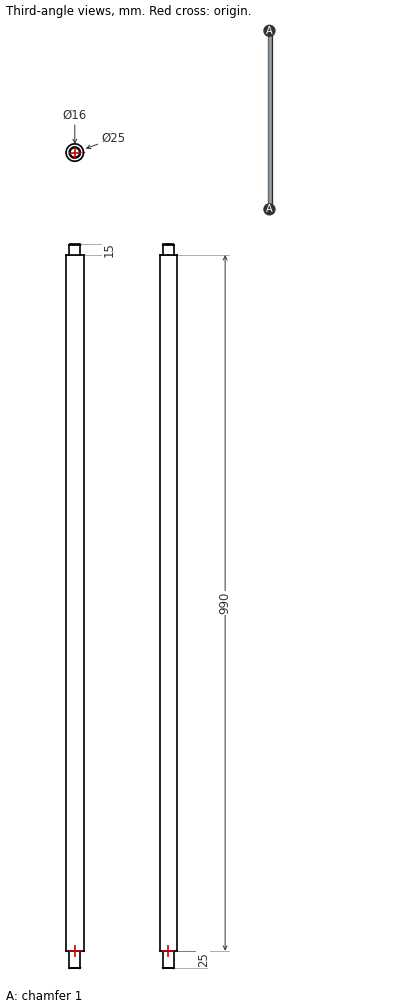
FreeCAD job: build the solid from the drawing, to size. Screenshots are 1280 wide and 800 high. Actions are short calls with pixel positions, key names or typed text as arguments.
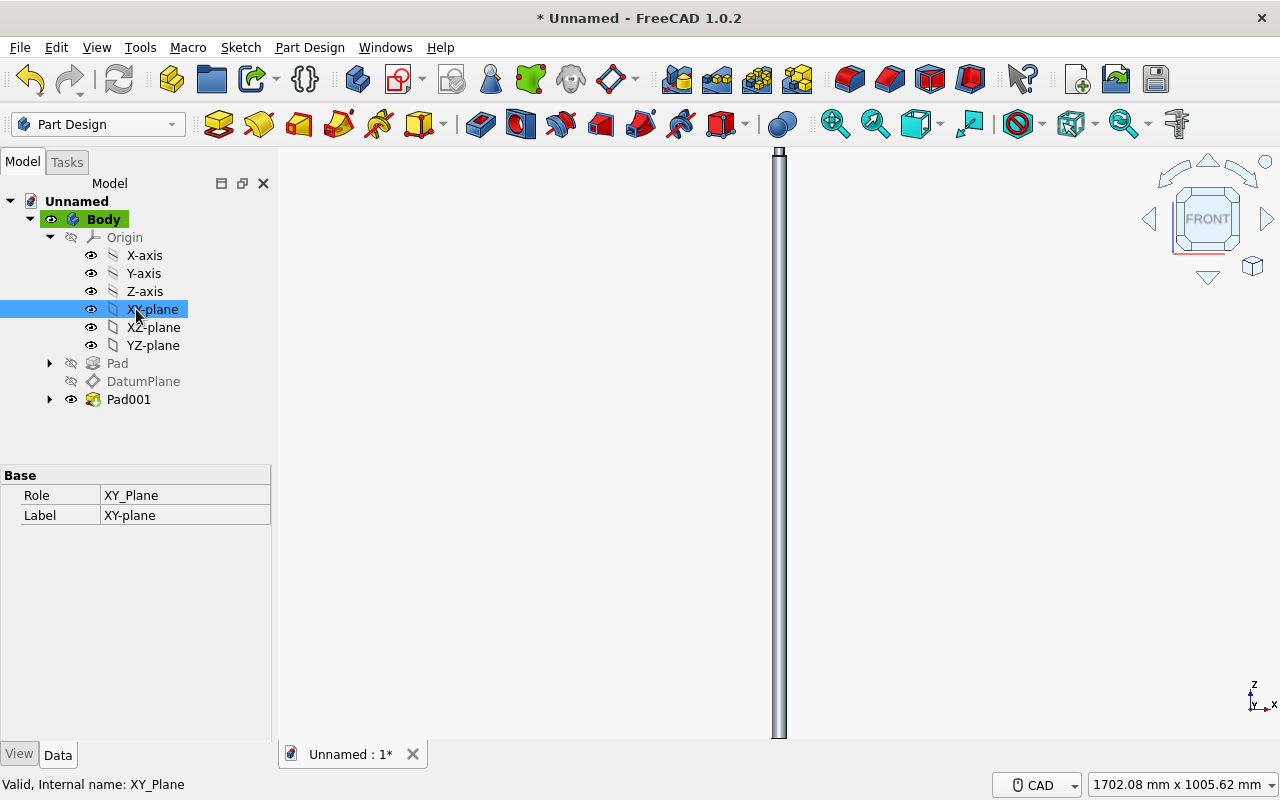
click(612, 80)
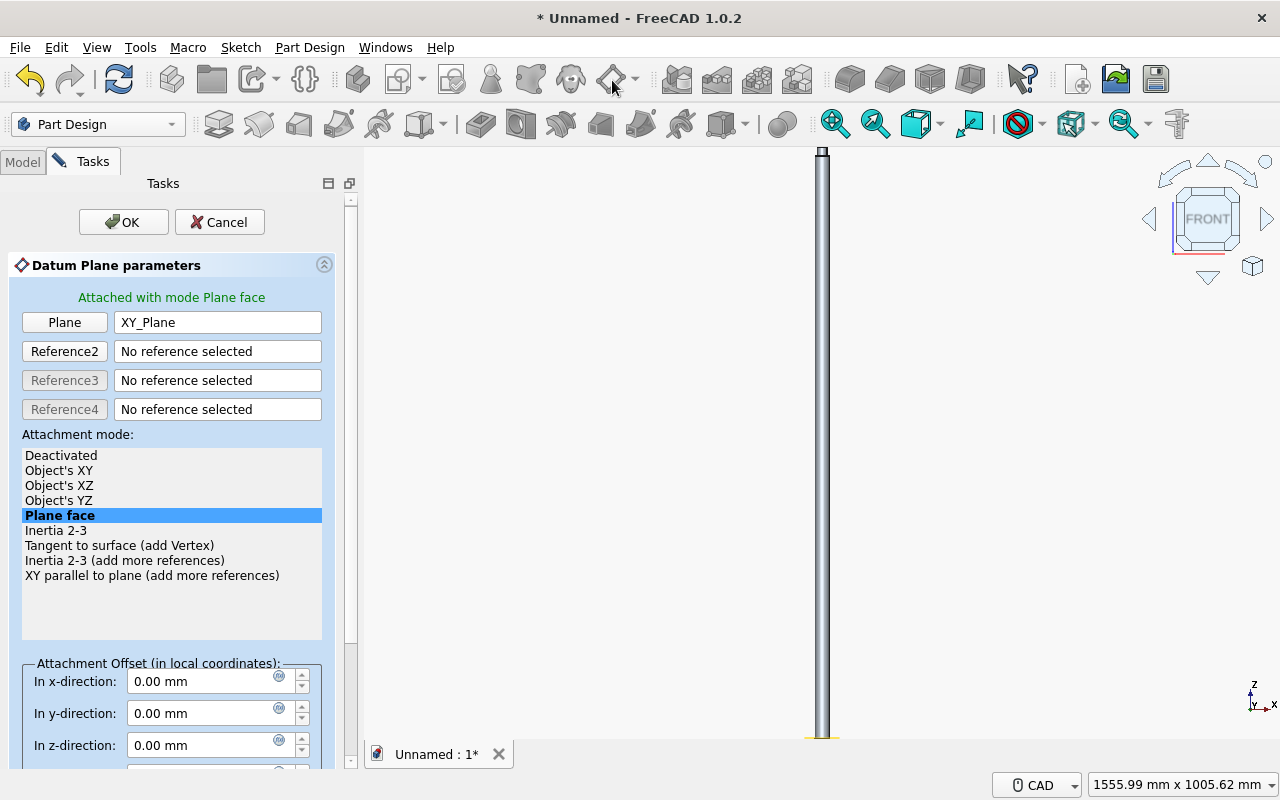
triple_click(210, 745)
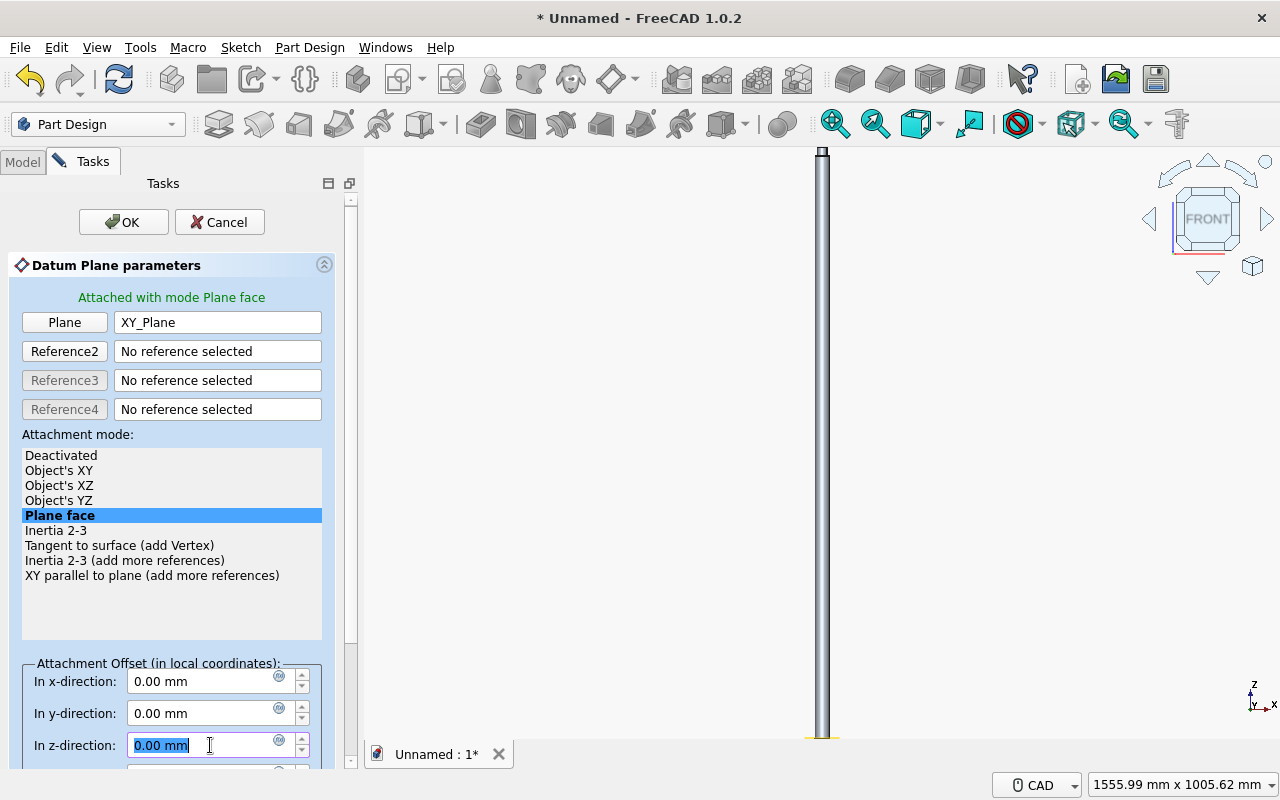
text(-25)
key(Tab)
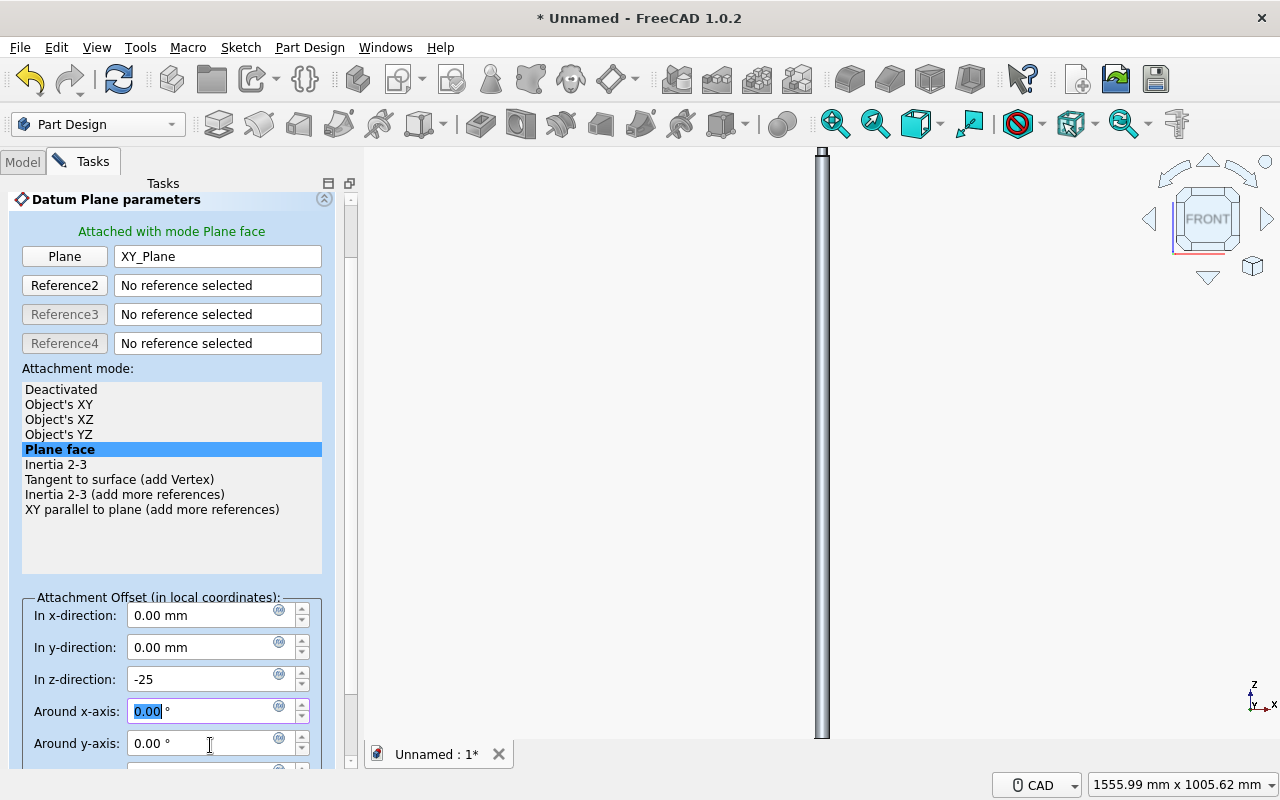
scroll(351, 480, up, 2)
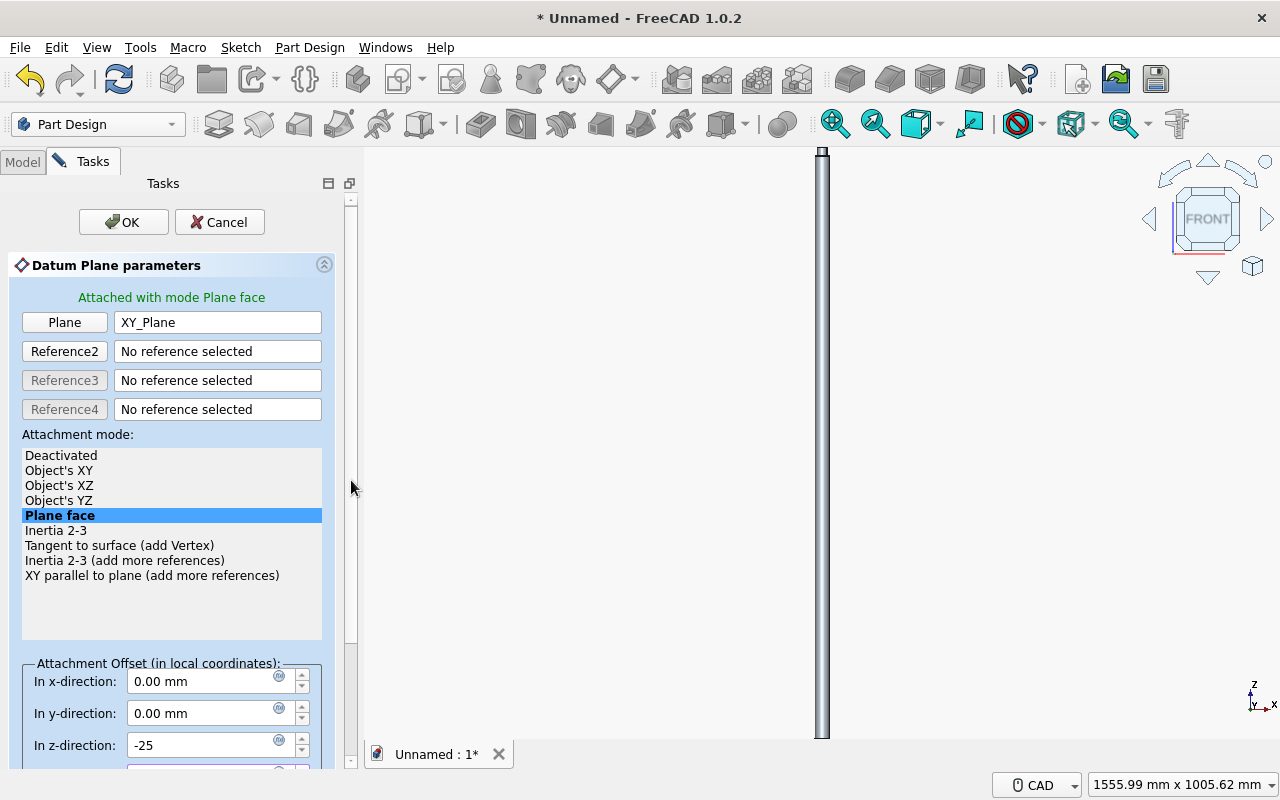
click(124, 222)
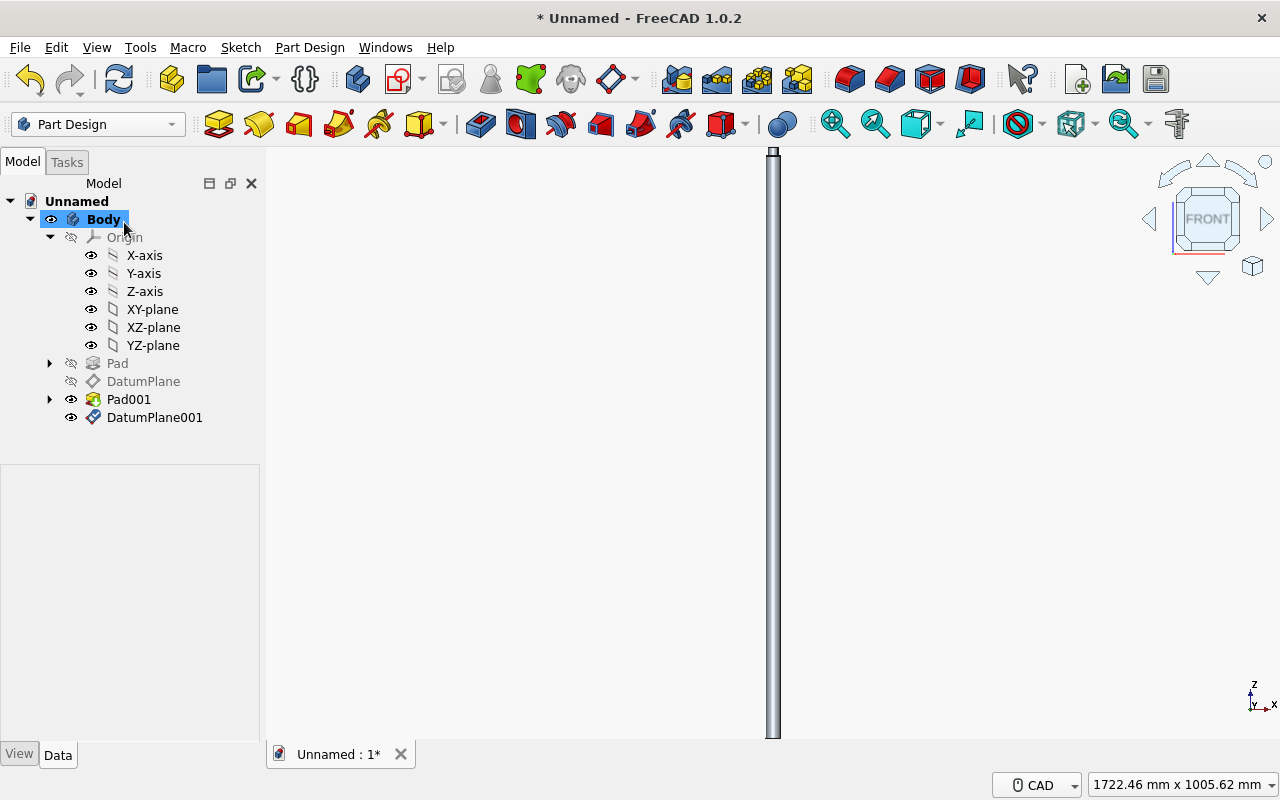
click(116, 417)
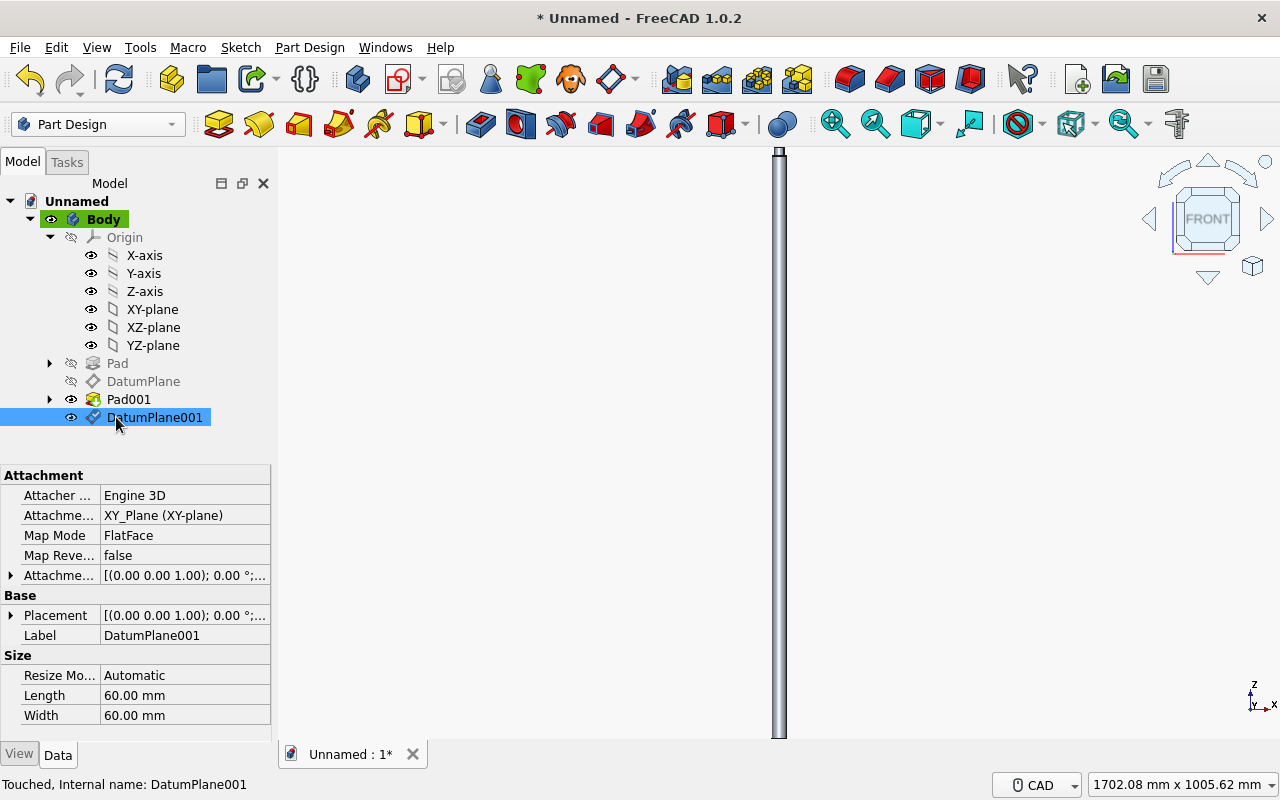
click(398, 80)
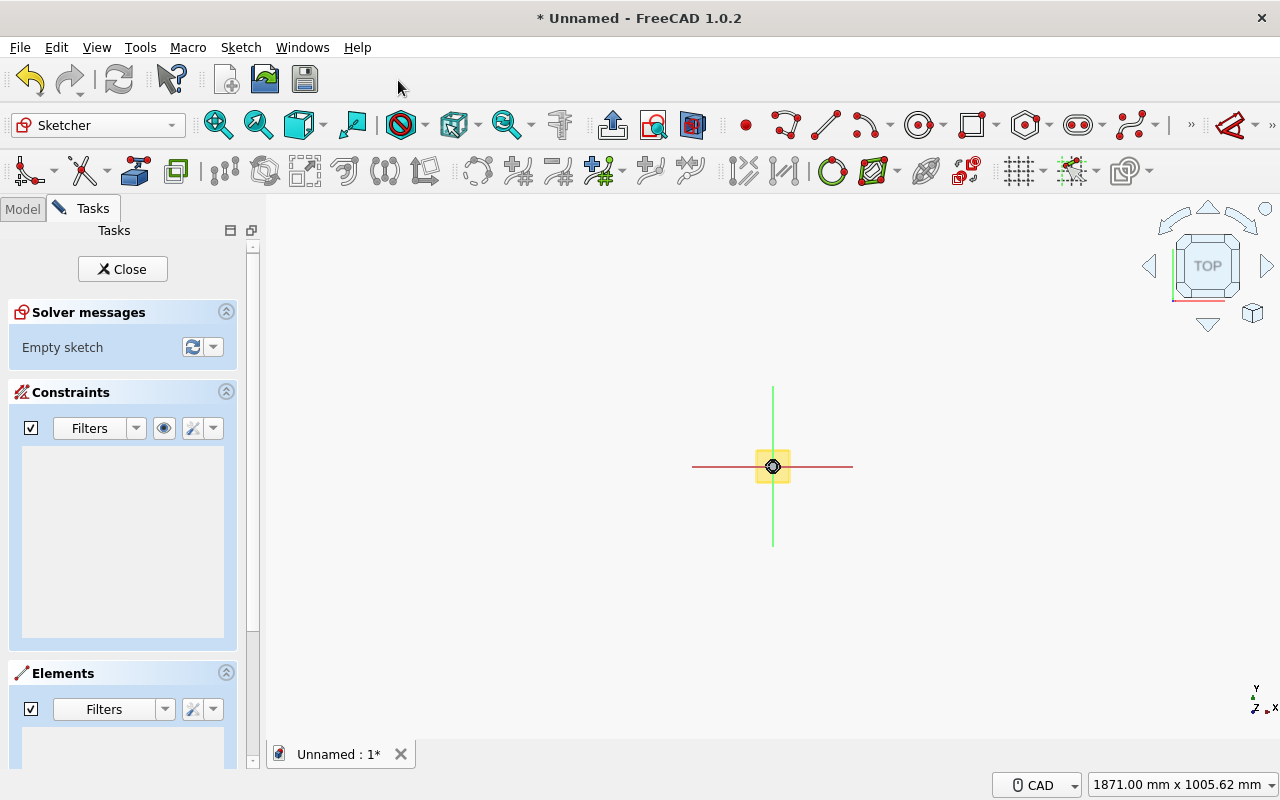
click(694, 126)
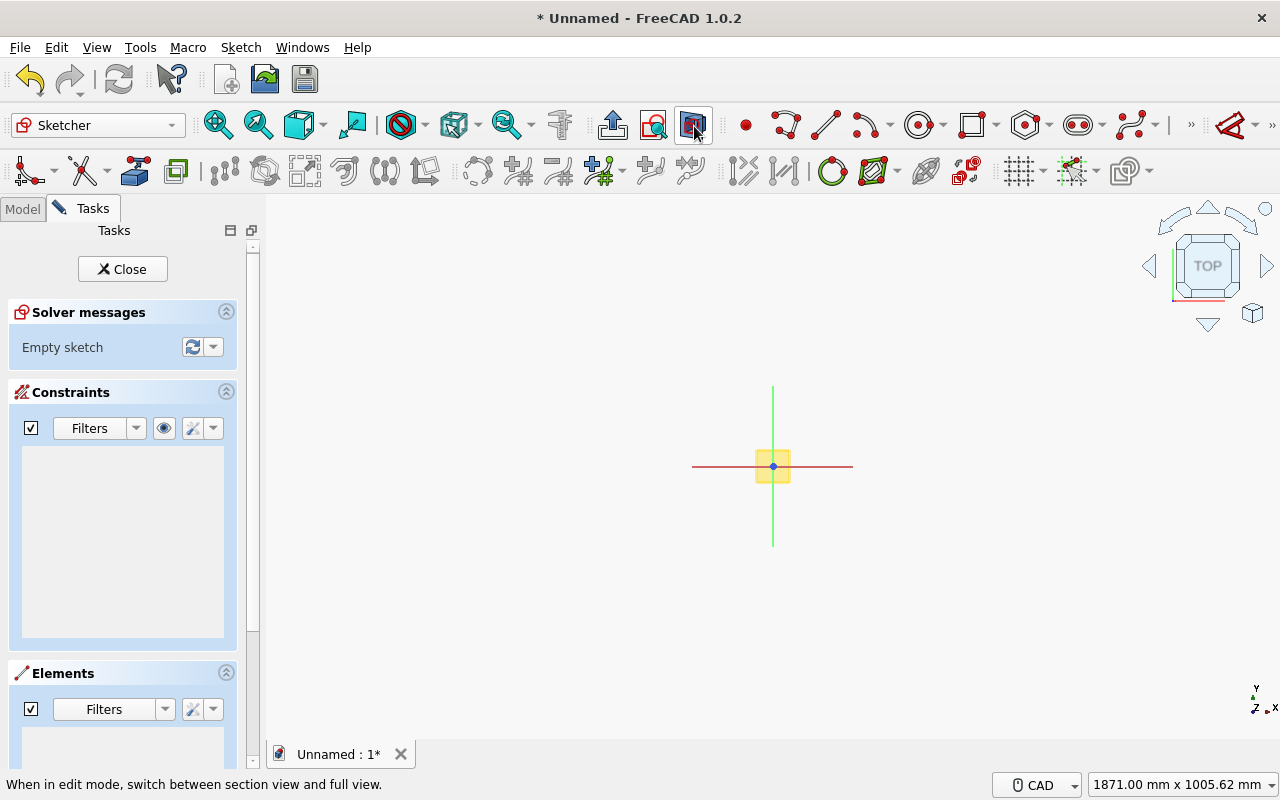
scroll(777, 466, up, 15)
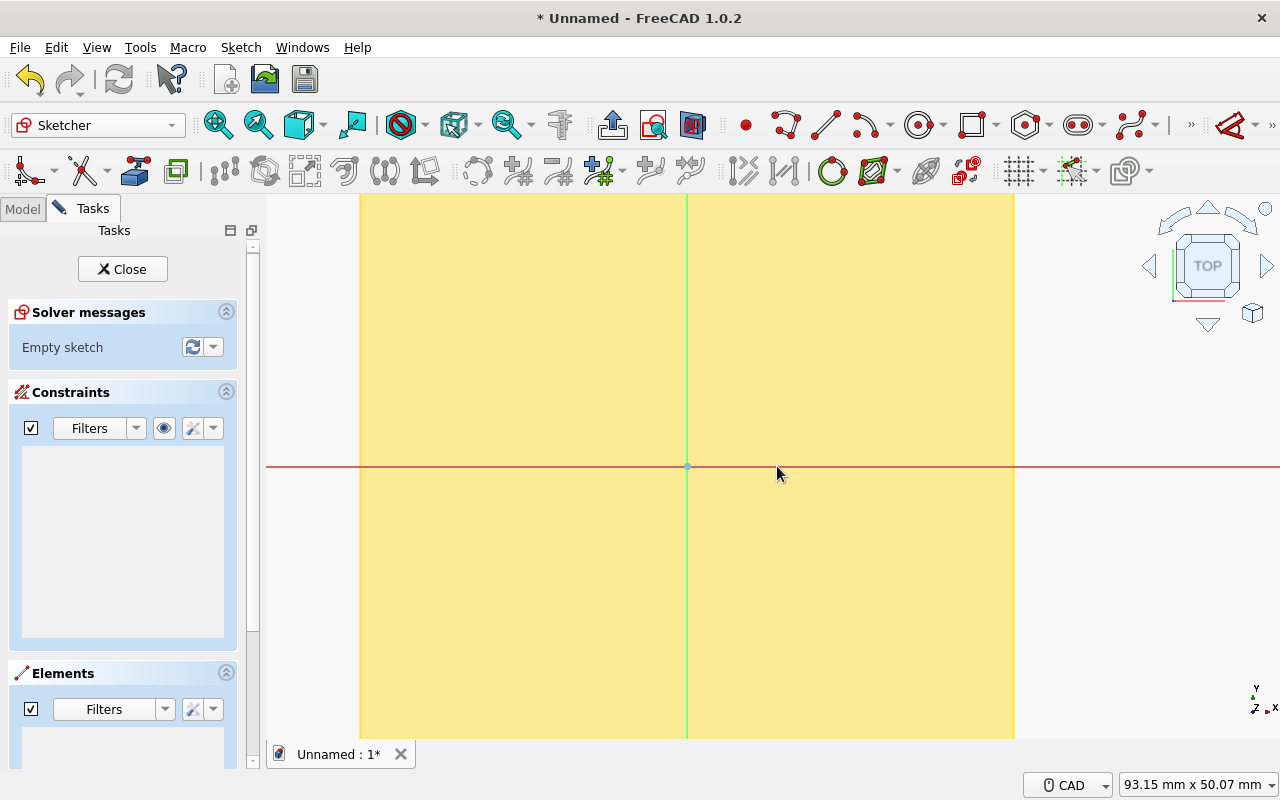
scroll(666, 466, up, 3)